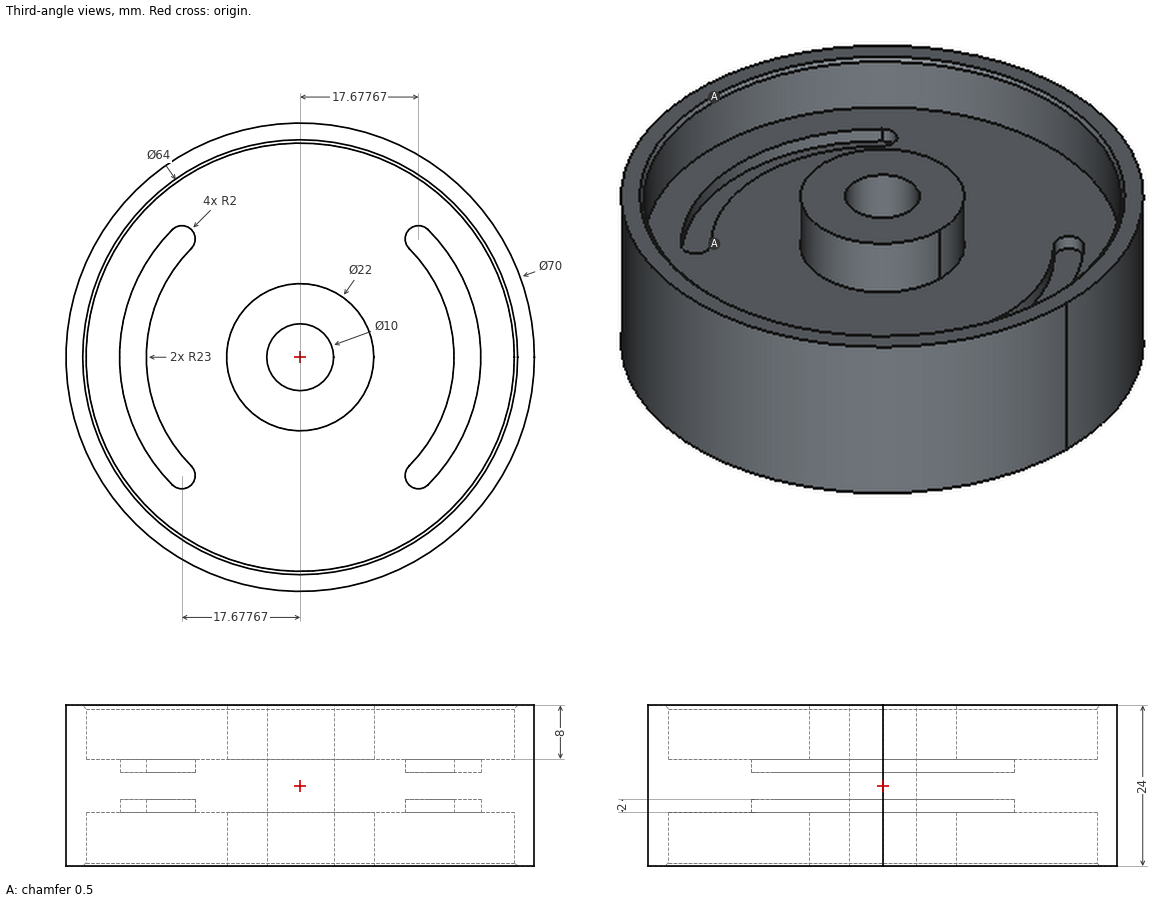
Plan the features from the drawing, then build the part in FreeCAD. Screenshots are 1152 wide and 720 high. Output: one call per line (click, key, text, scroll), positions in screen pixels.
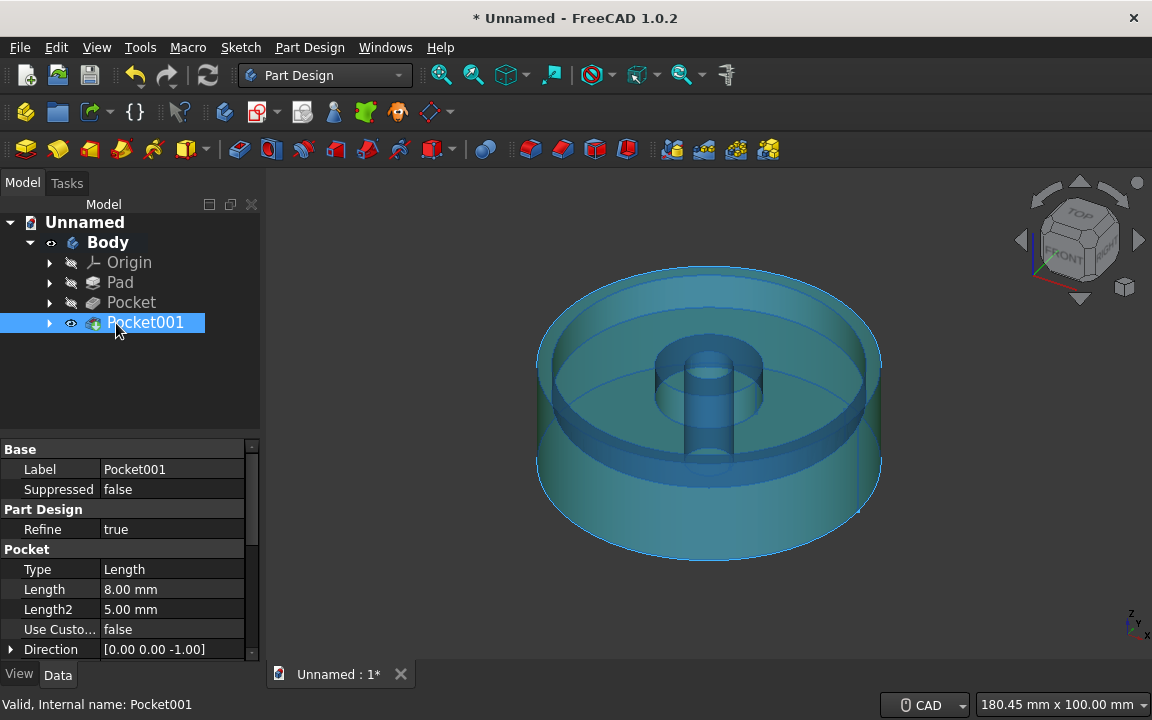
click(672, 150)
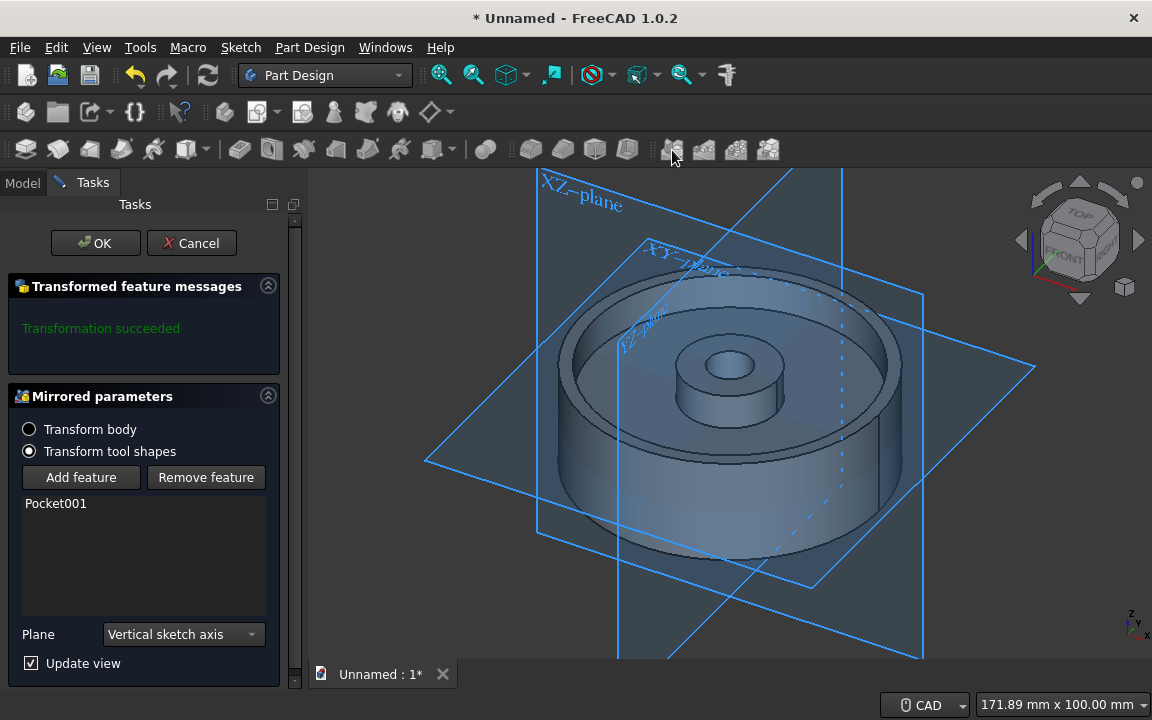
click(184, 634)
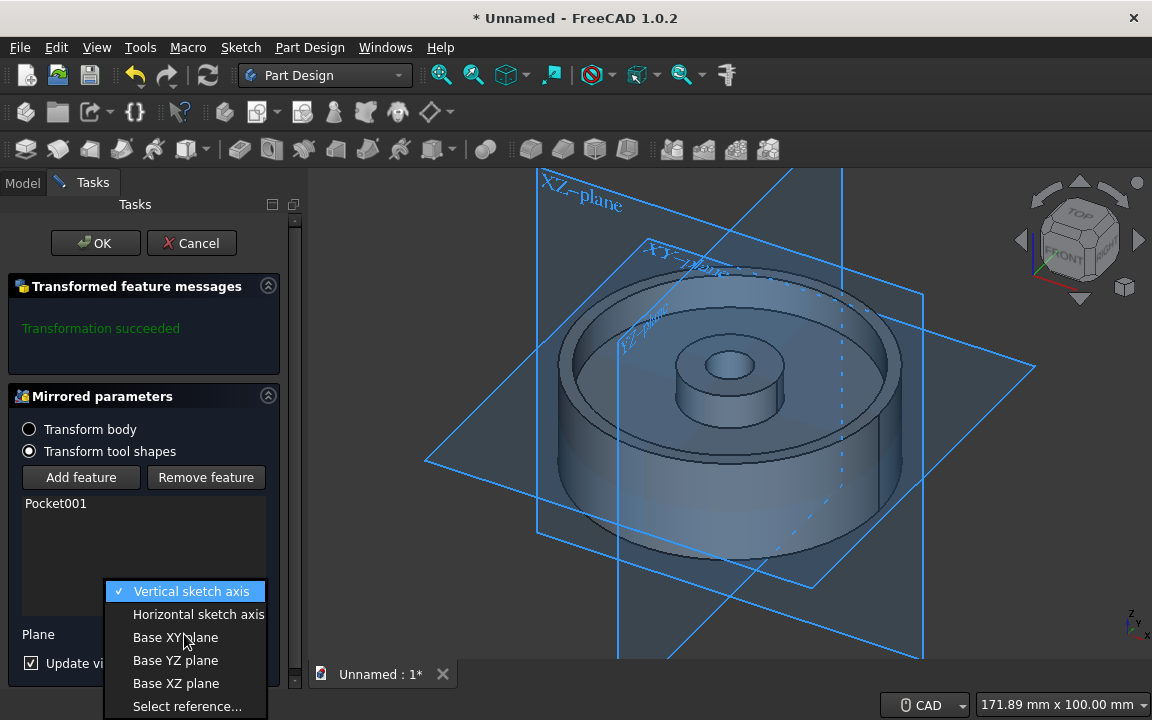
click(184, 638)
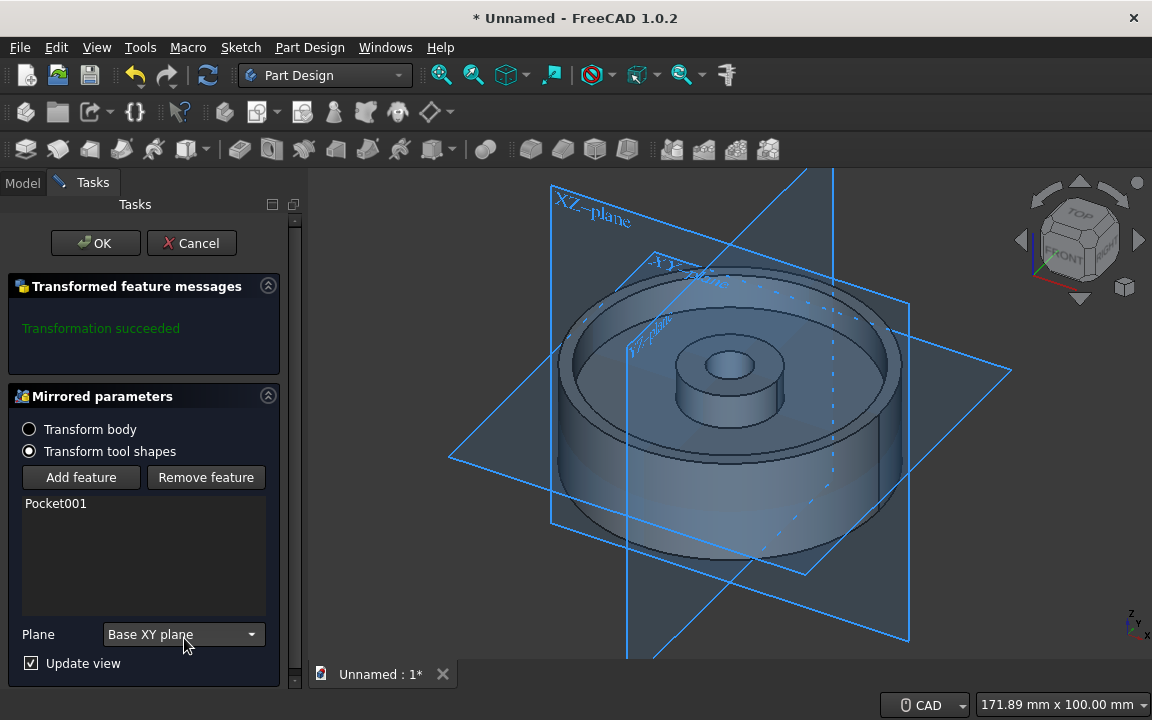
click(96, 243)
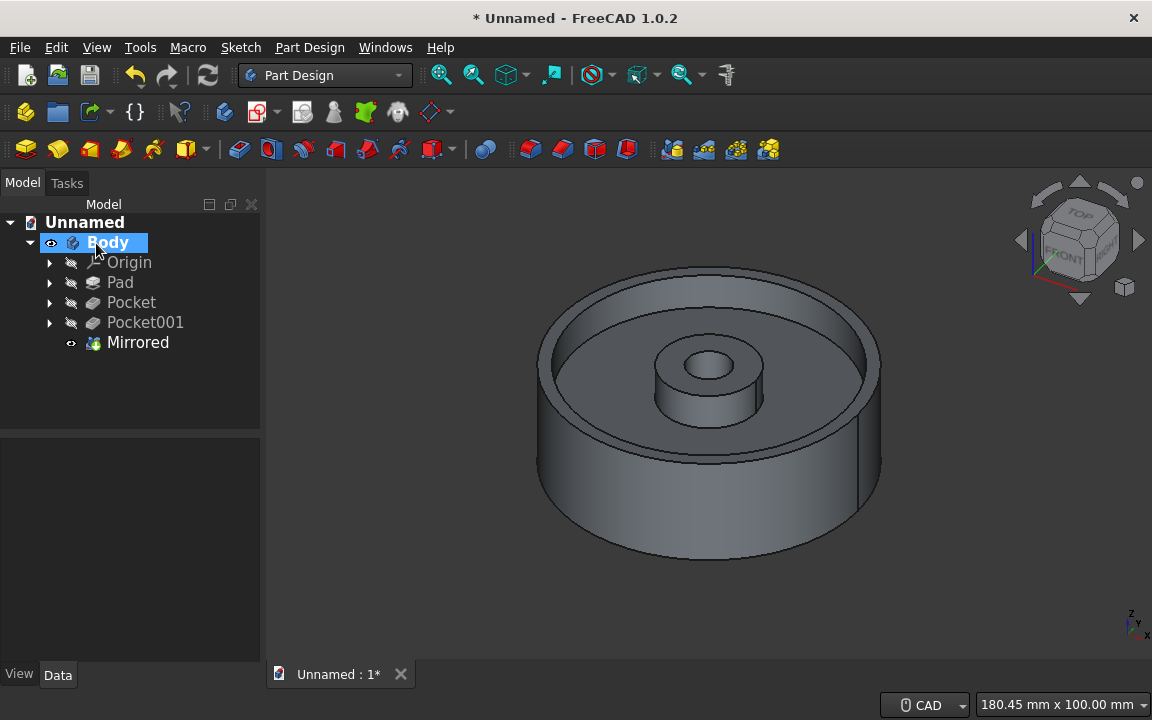
key(5)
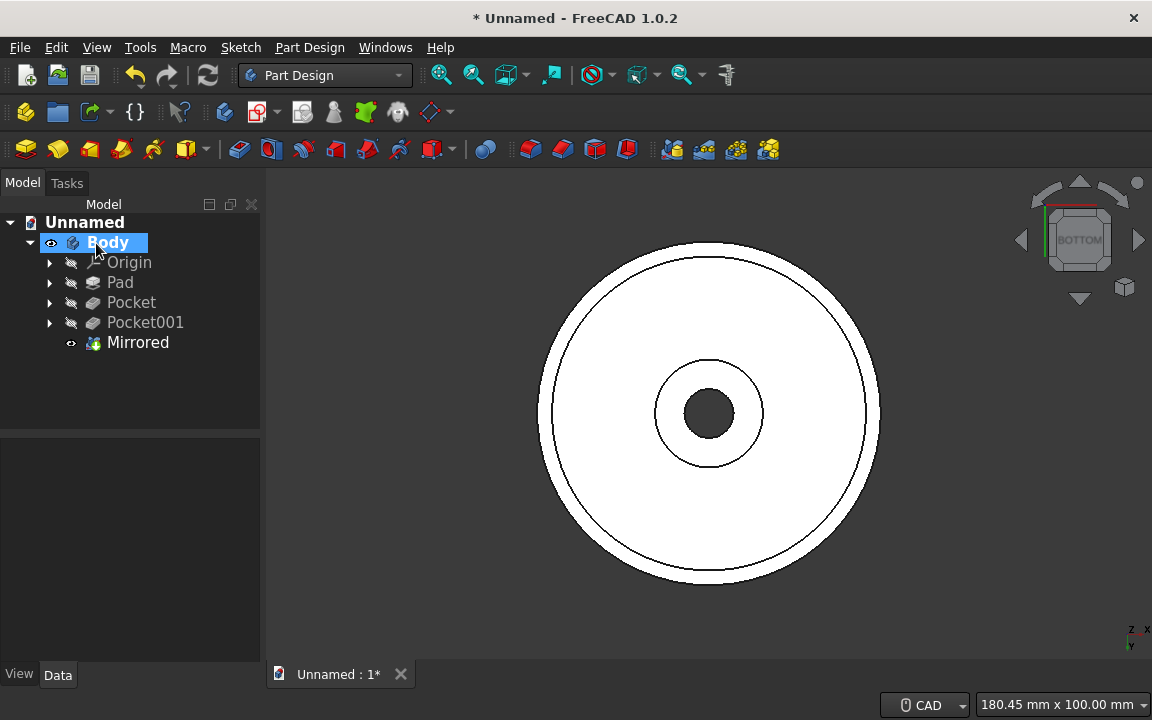
click(799, 457)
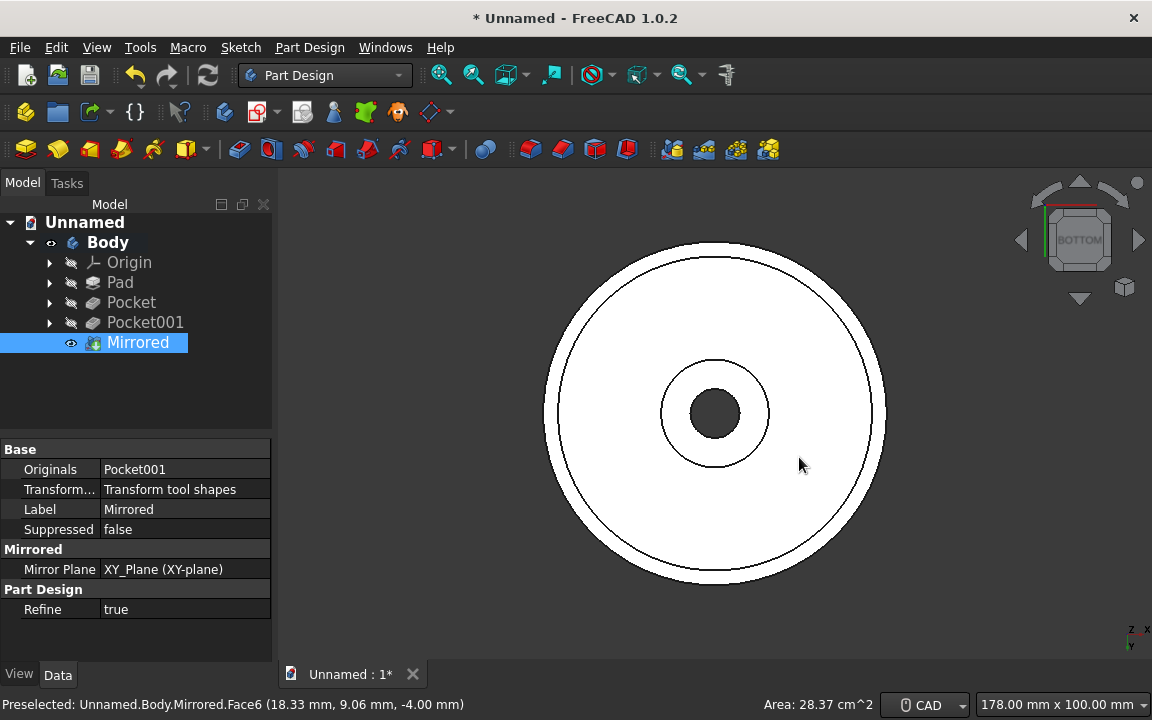
click(258, 112)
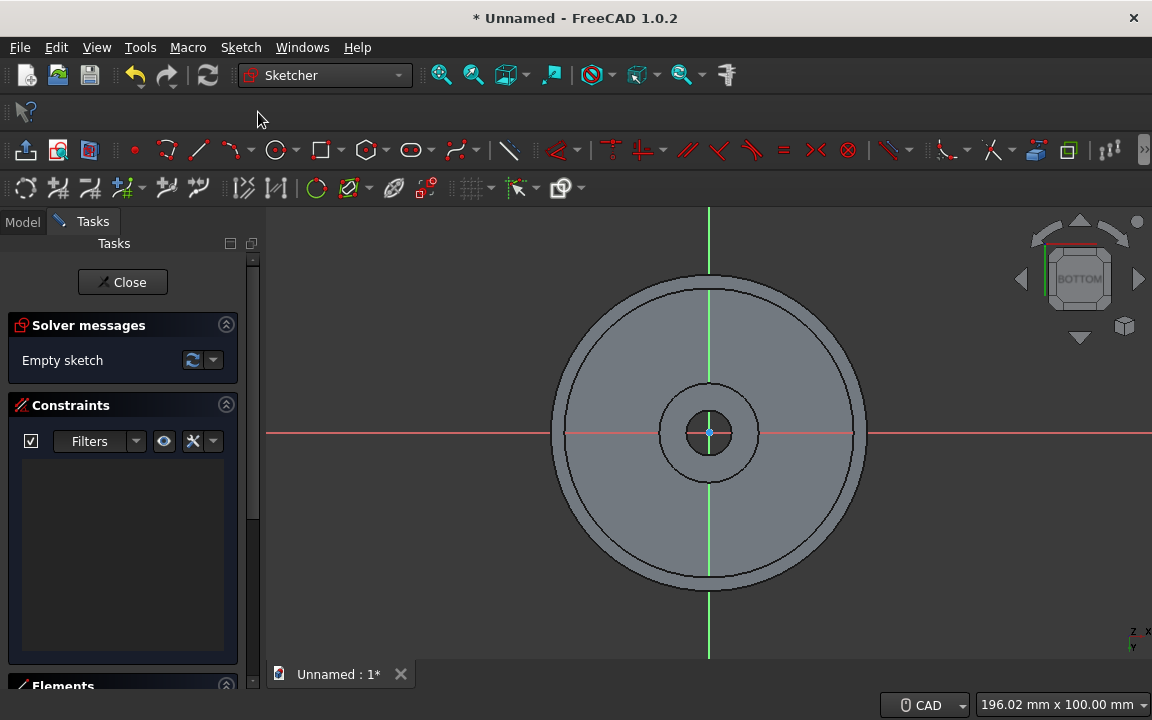
scroll(848, 433, up, 2)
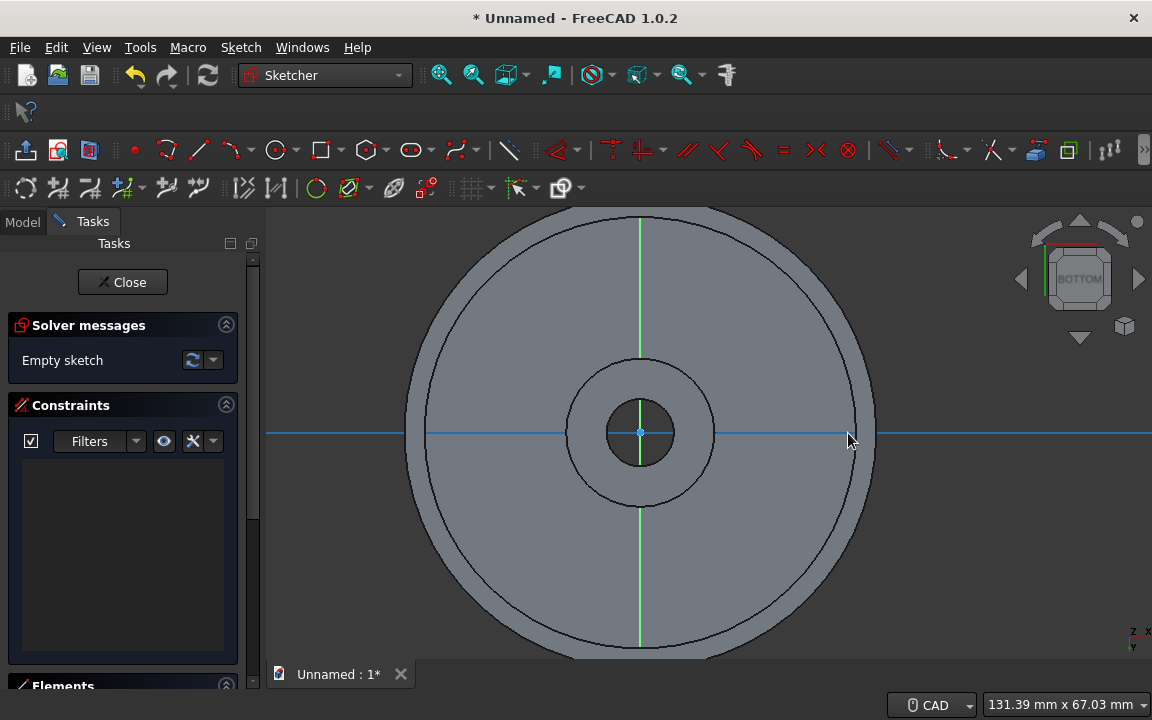
key(g)
key(3)
key(a)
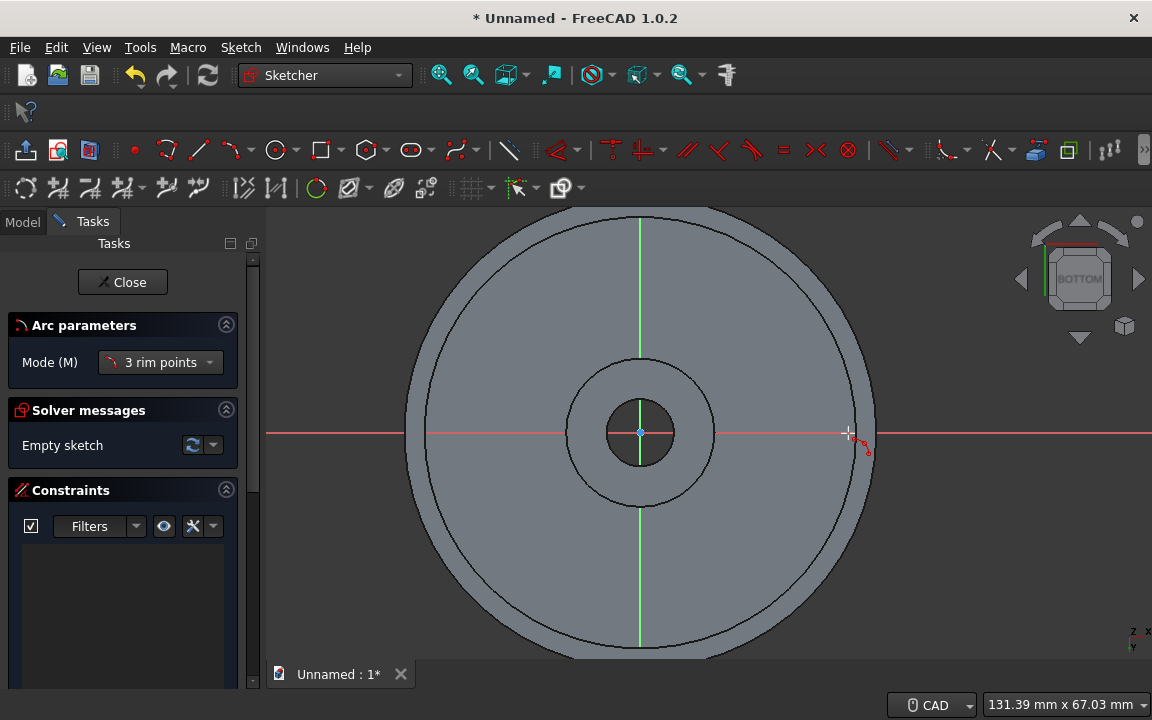
click(531, 542)
click(531, 323)
click(487, 408)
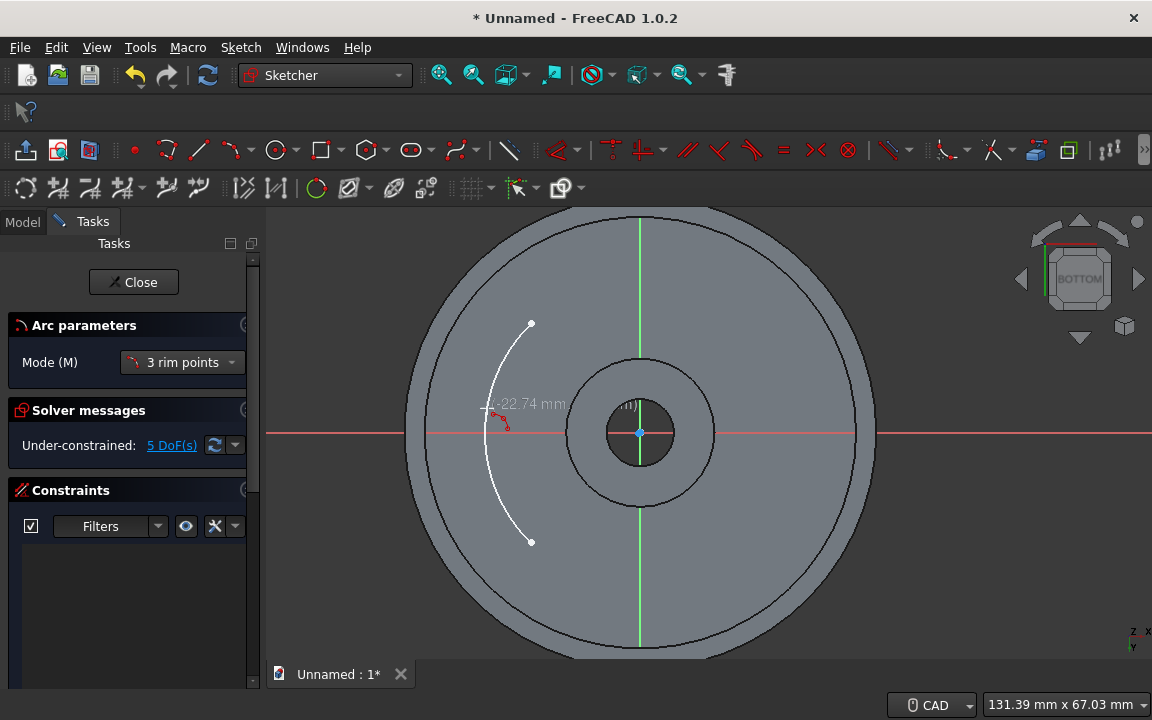
click(531, 324)
click(512, 304)
click(531, 304)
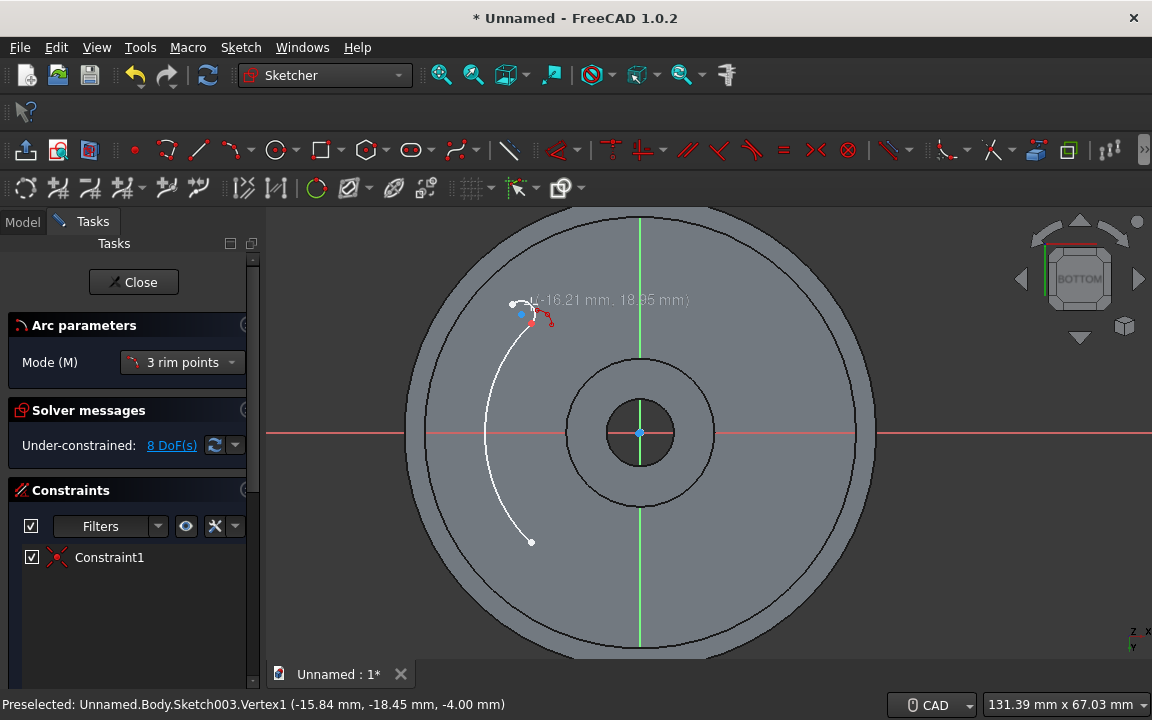
click(512, 305)
click(512, 561)
click(460, 404)